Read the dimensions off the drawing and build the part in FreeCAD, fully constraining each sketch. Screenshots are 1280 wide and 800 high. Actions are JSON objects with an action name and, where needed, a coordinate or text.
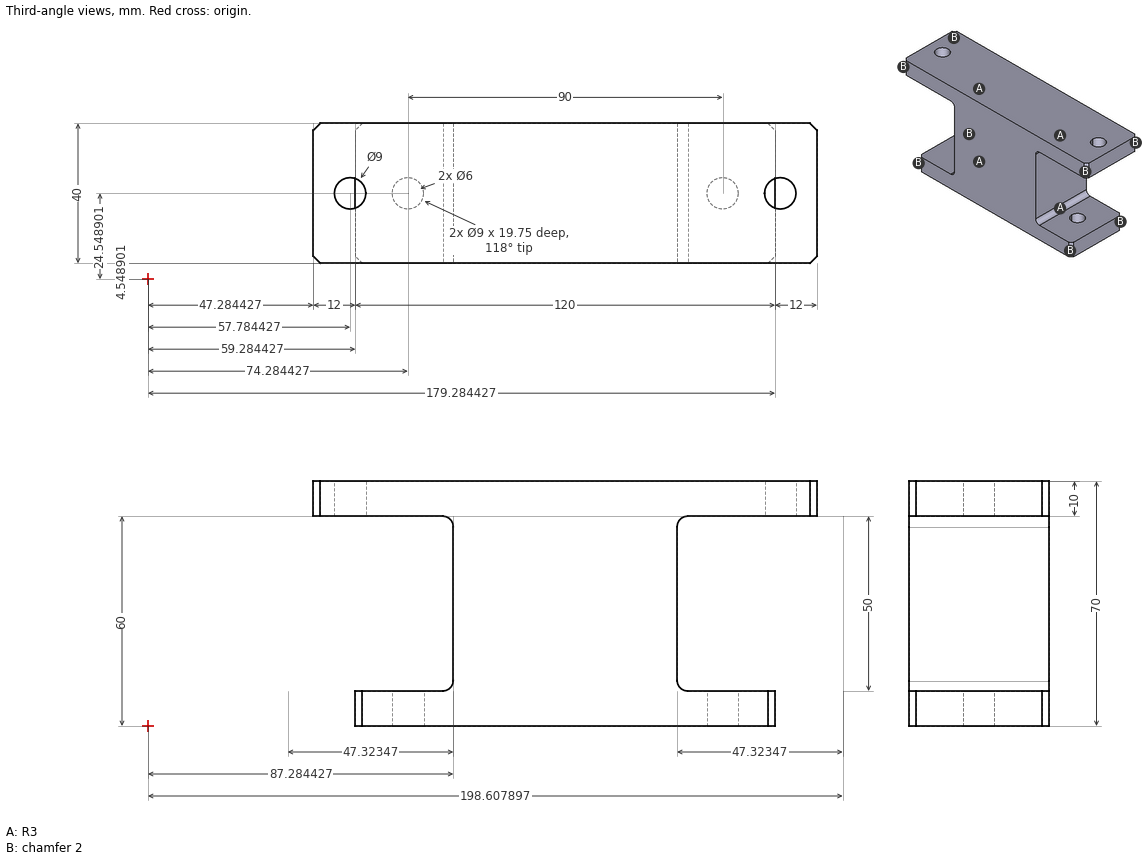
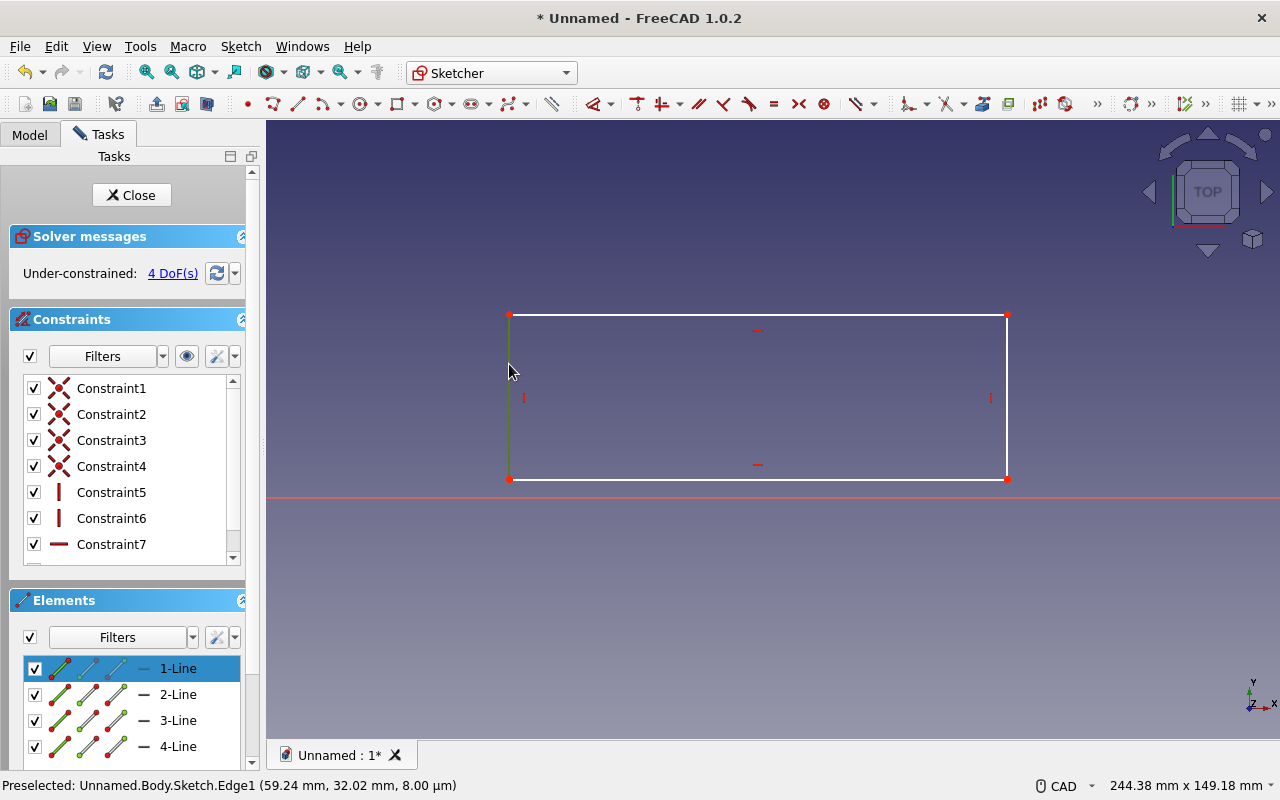
{"action": "left_click", "coordinate": [610, 104]}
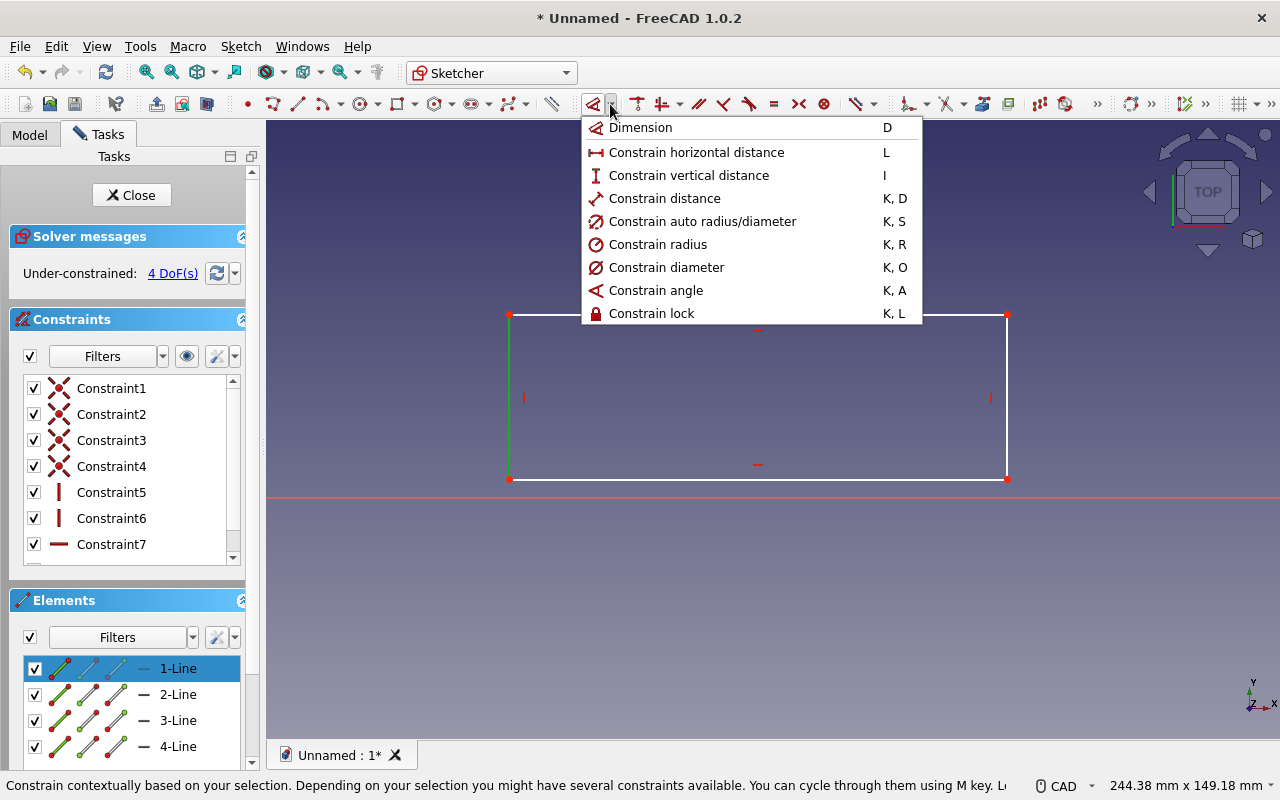
{"action": "left_click", "coordinate": [752, 176]}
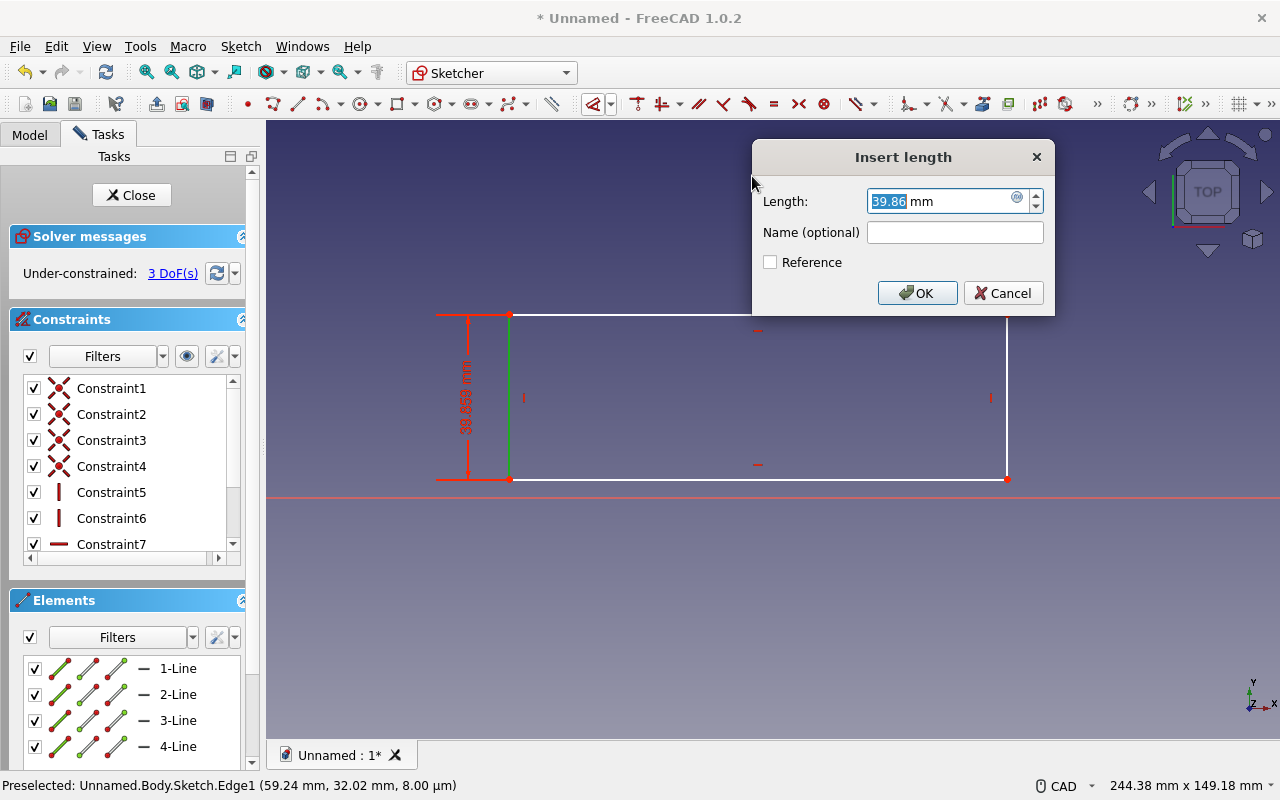
{"action": "type", "text": "40"}
{"action": "key", "text": "Return"}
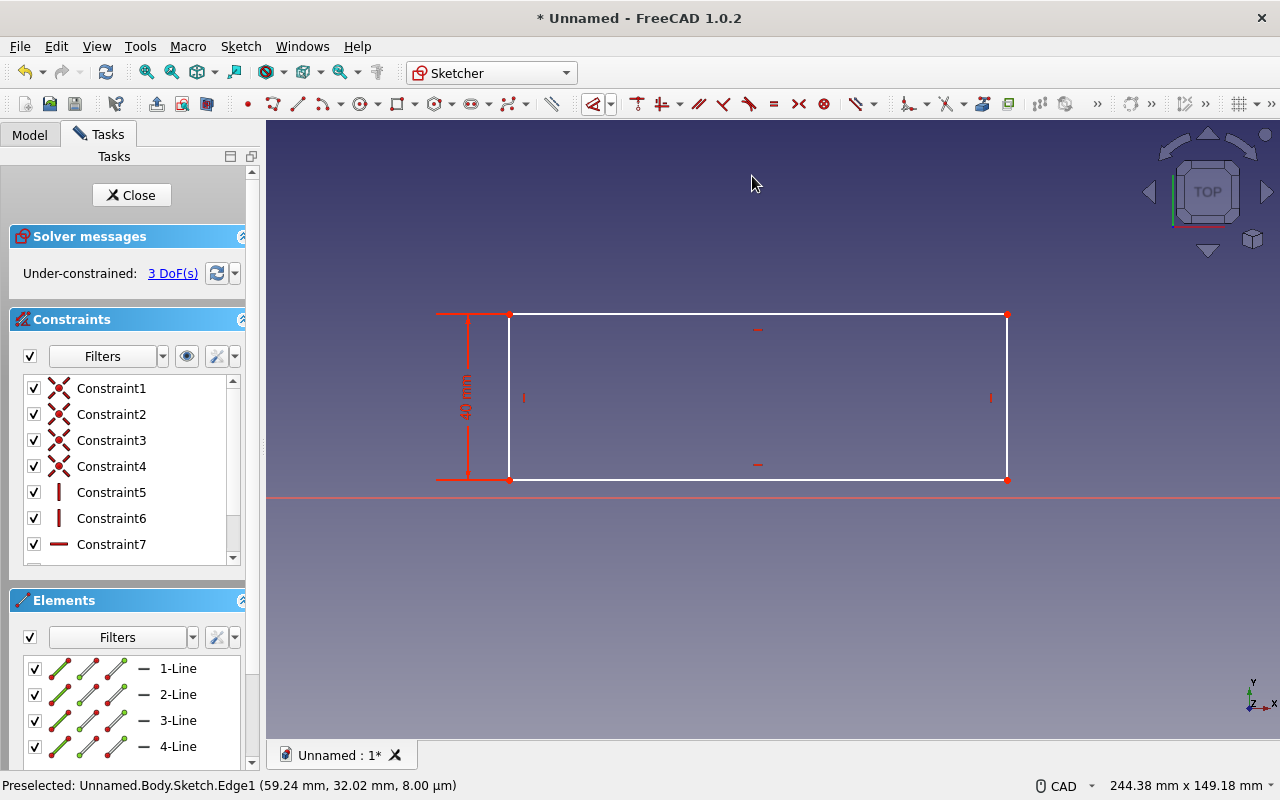
{"action": "left_click", "coordinate": [659, 480]}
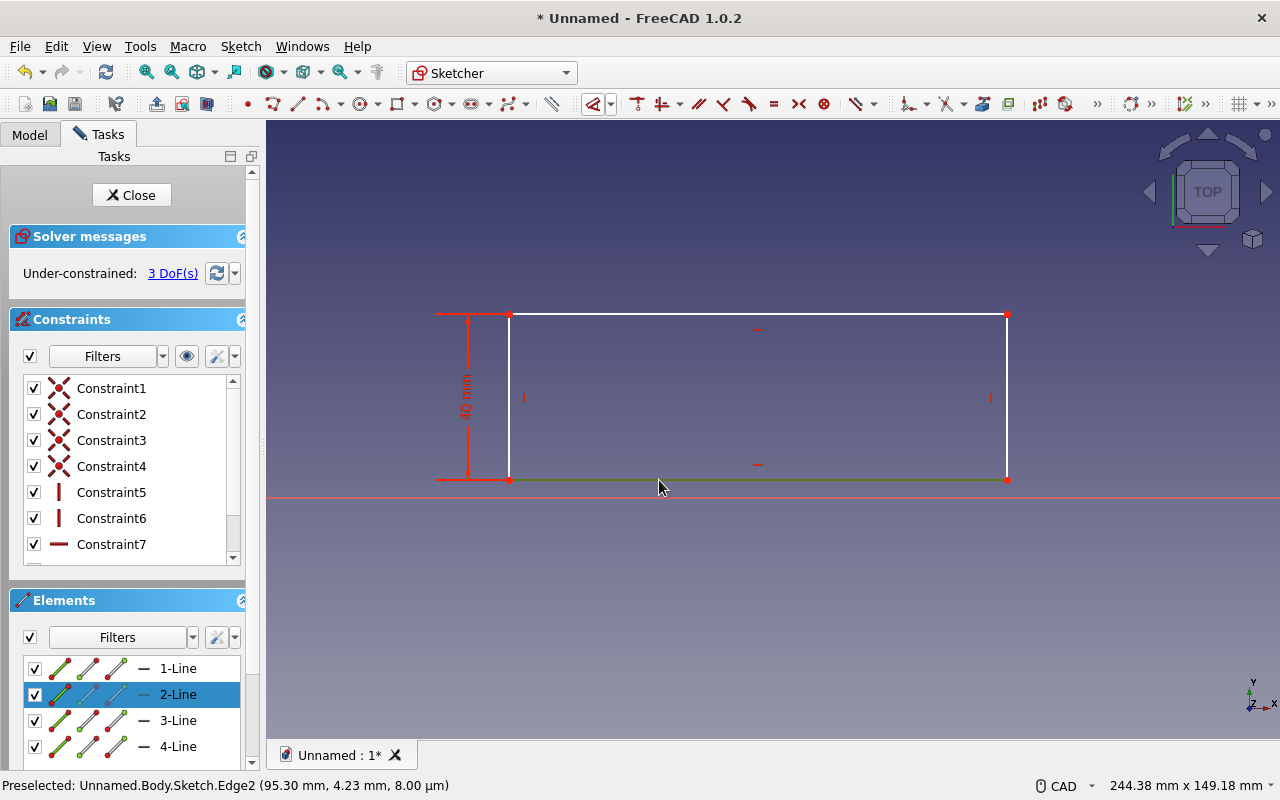
{"action": "key", "text": "l"}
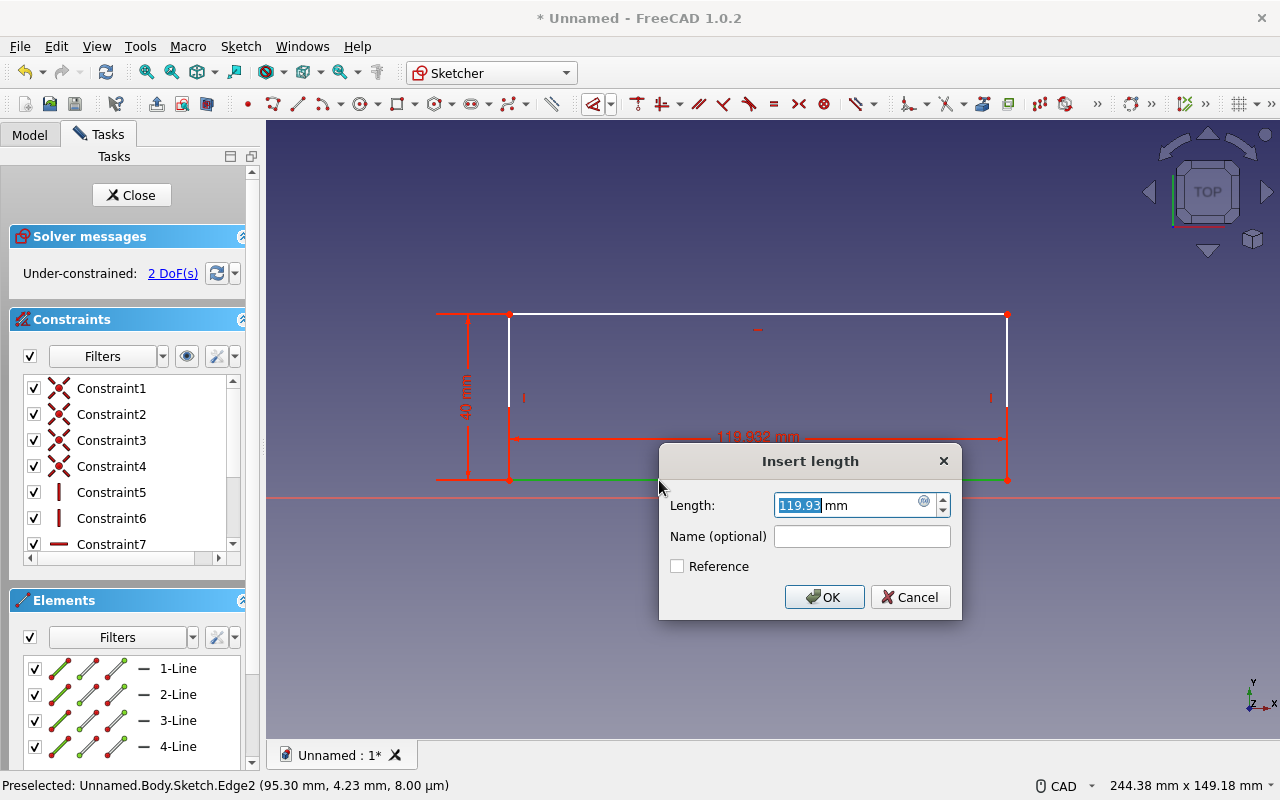
{"action": "type", "text": "120"}
{"action": "key", "text": "Return"}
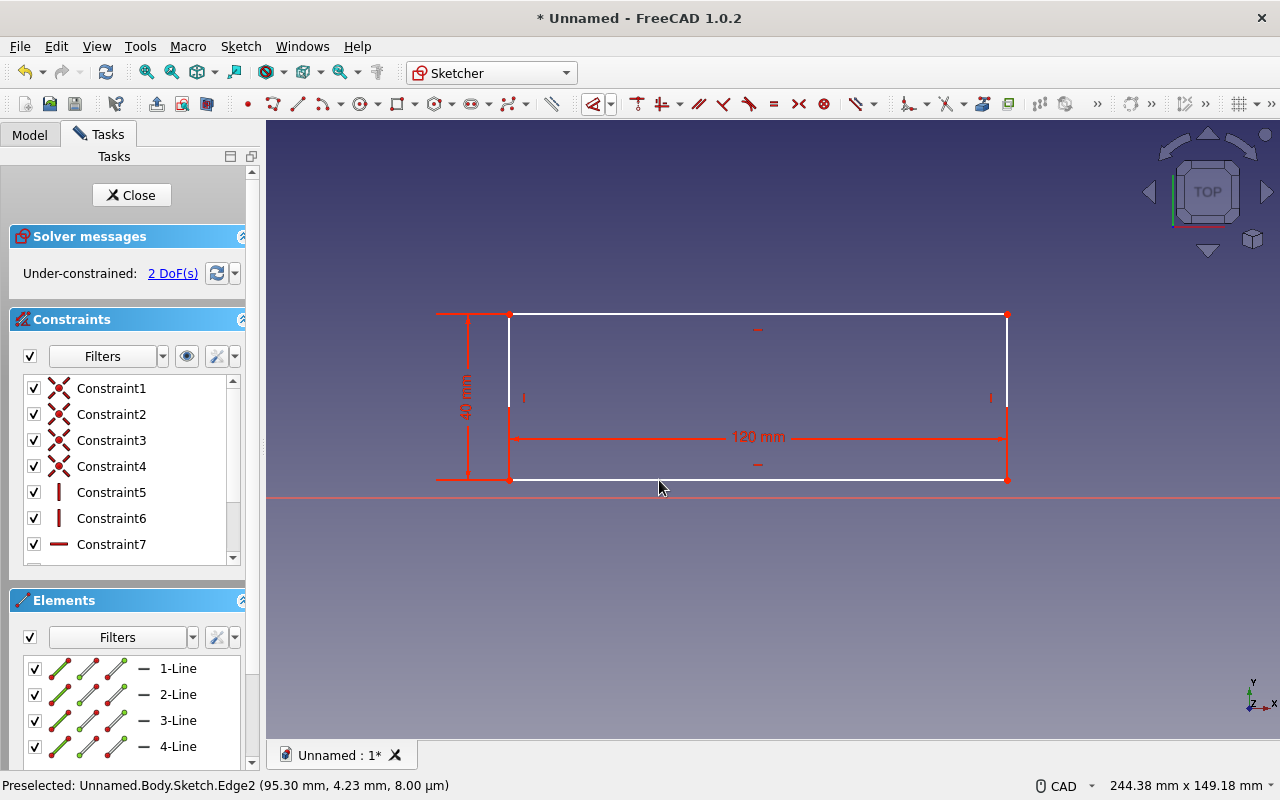
{"action": "scroll", "coordinate": [509, 480], "scroll_direction": "up", "scroll_amount": 4}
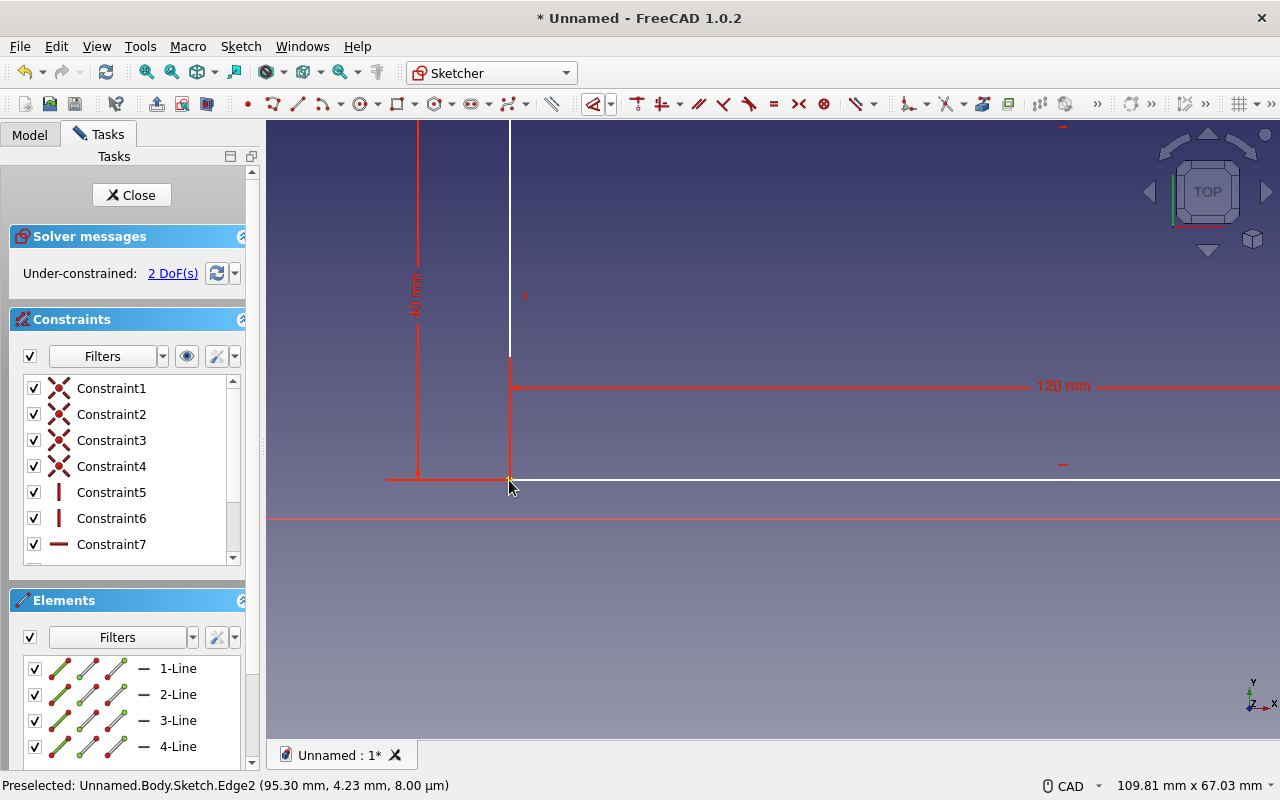
{"action": "left_click", "coordinate": [510, 480]}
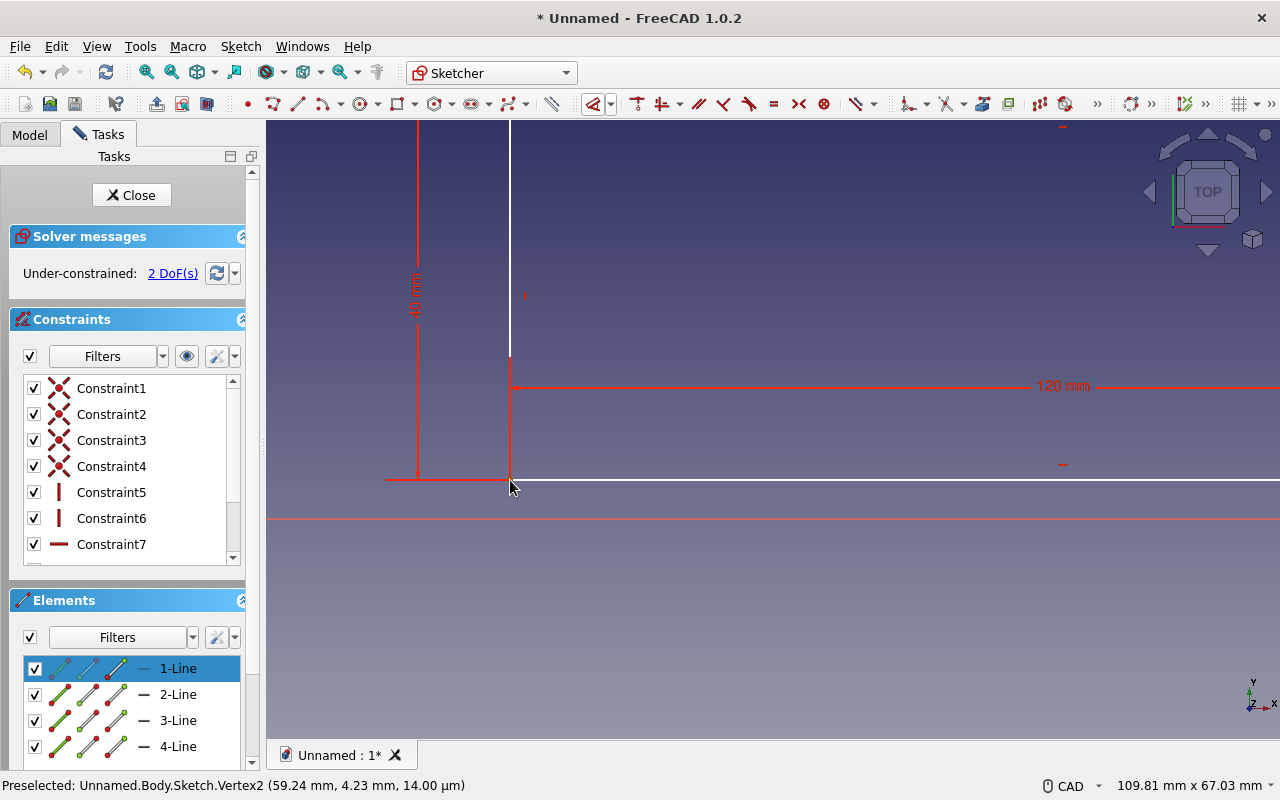
{"action": "left_click", "coordinate": [610, 104]}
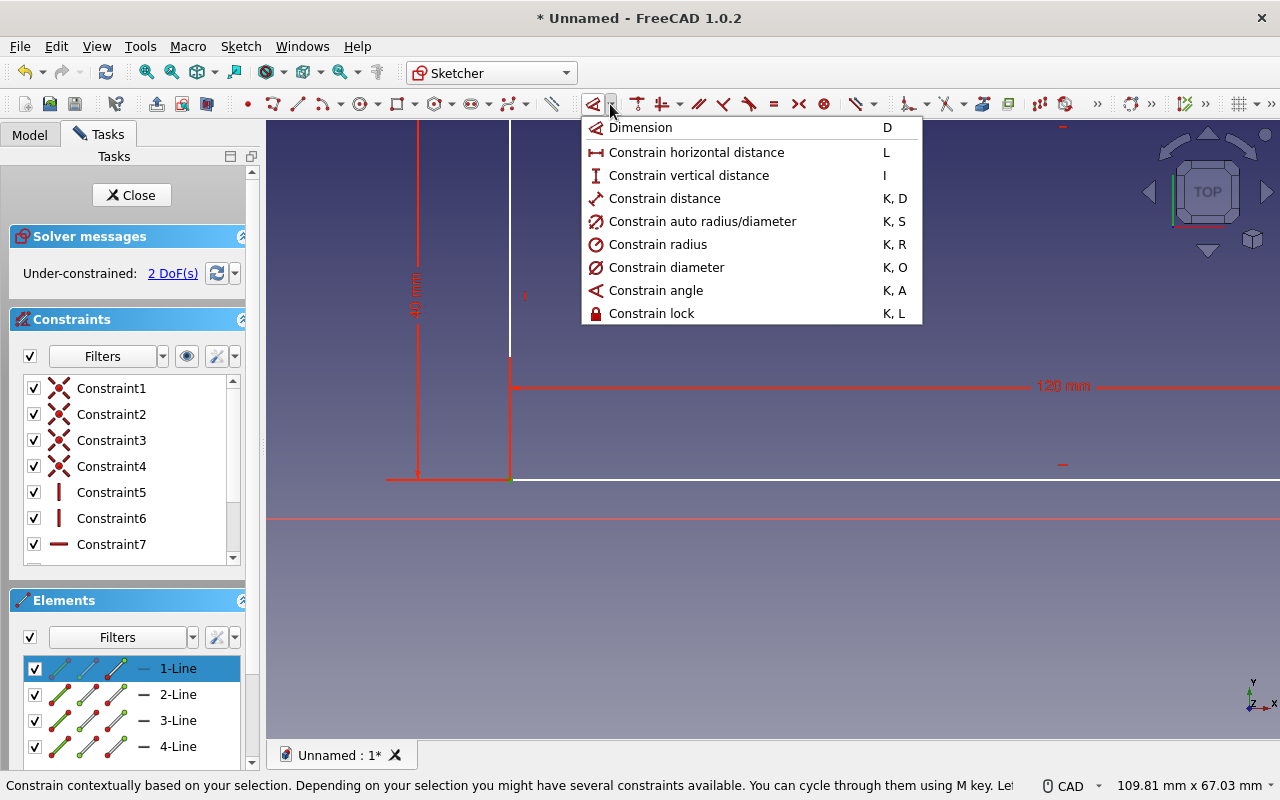
{"action": "left_click", "coordinate": [752, 176]}